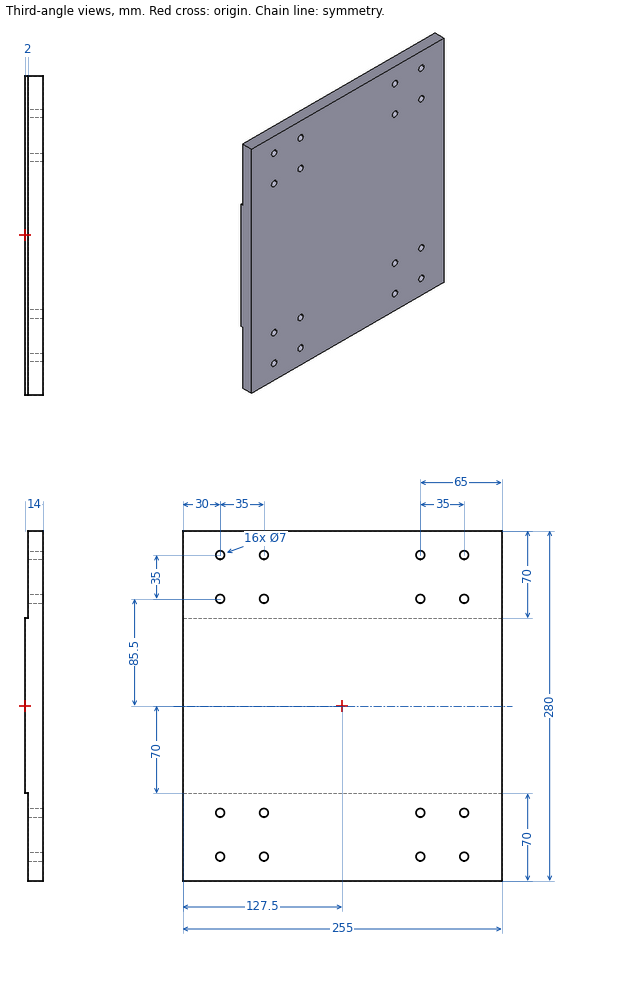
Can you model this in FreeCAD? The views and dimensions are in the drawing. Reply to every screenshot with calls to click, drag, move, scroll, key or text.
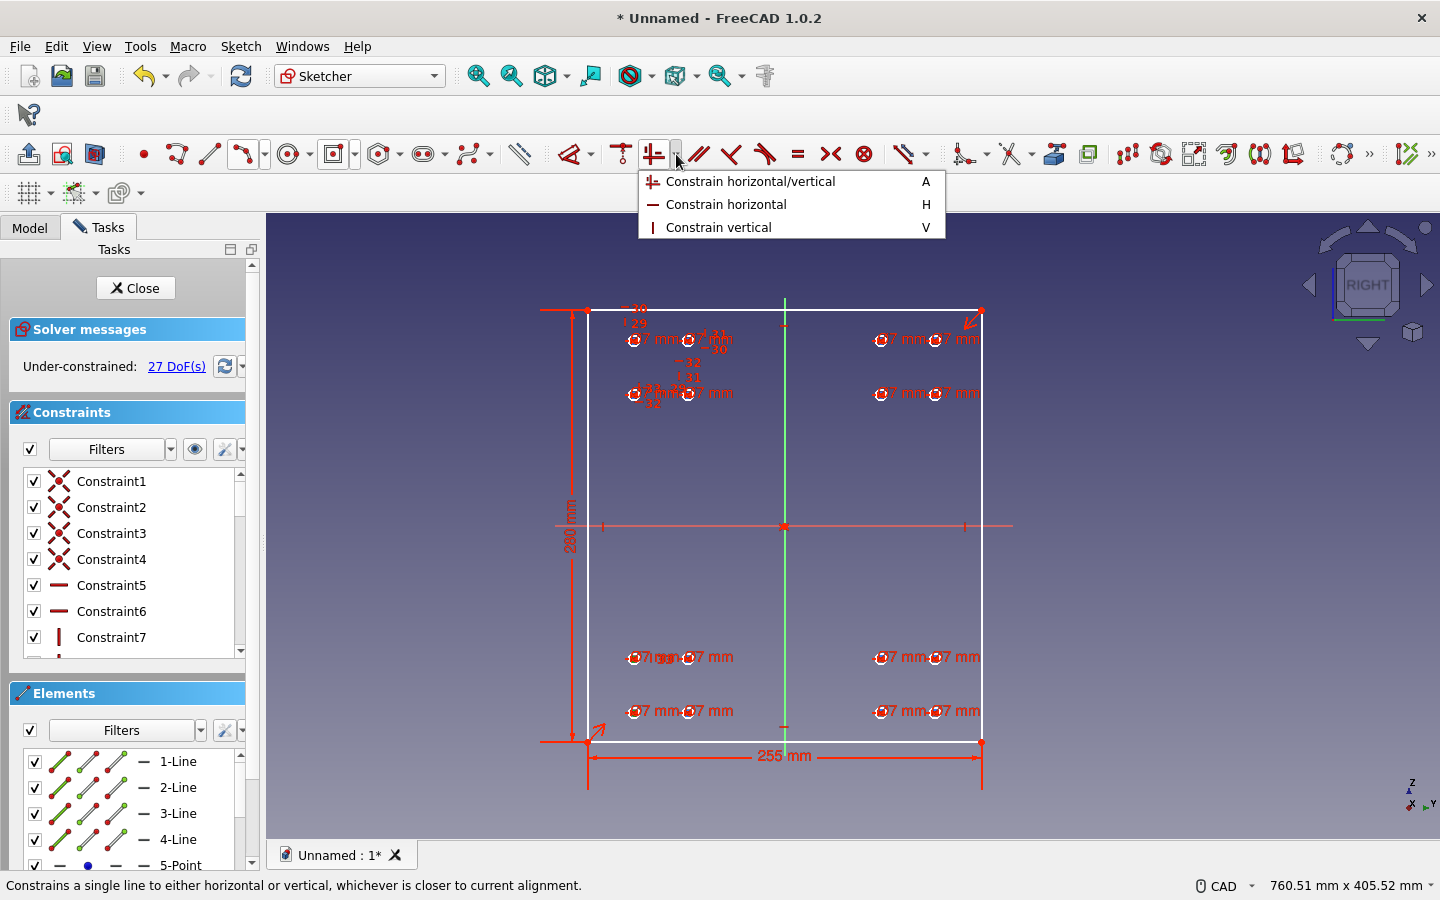
click(792, 228)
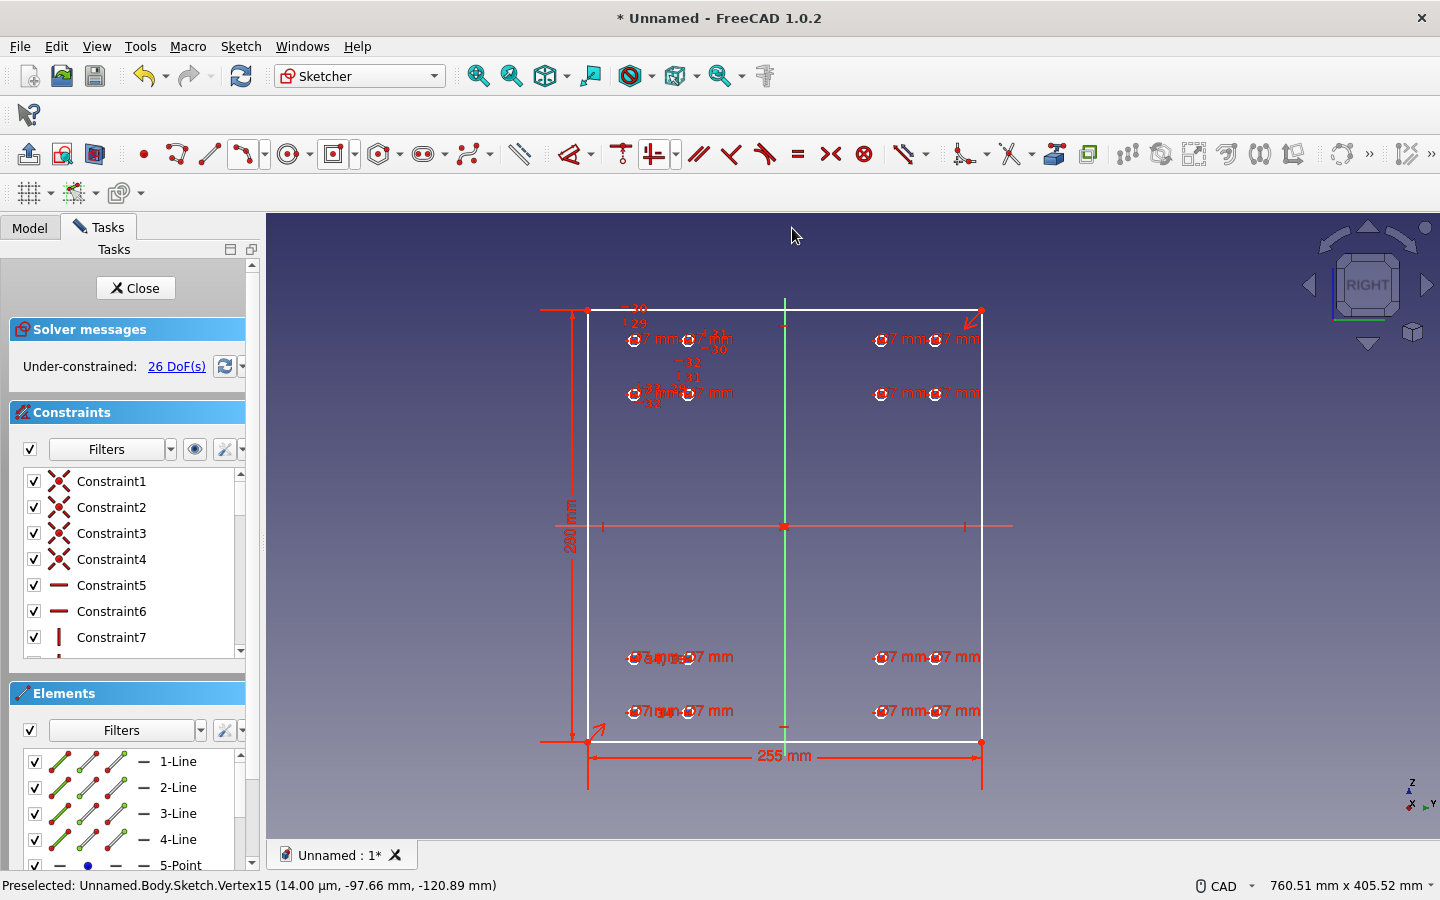
click(688, 395)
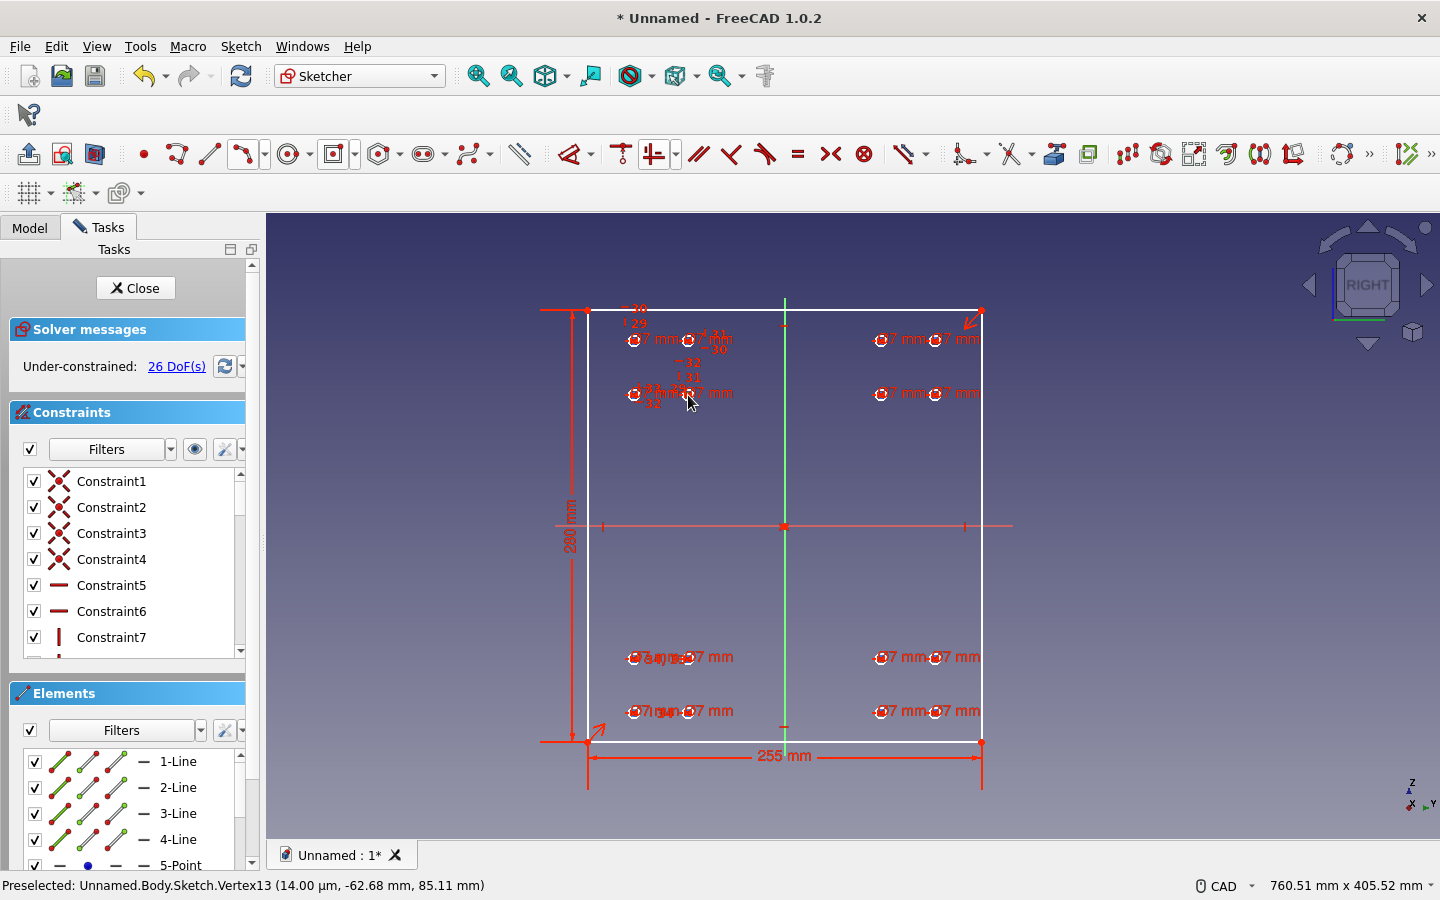
click(688, 659)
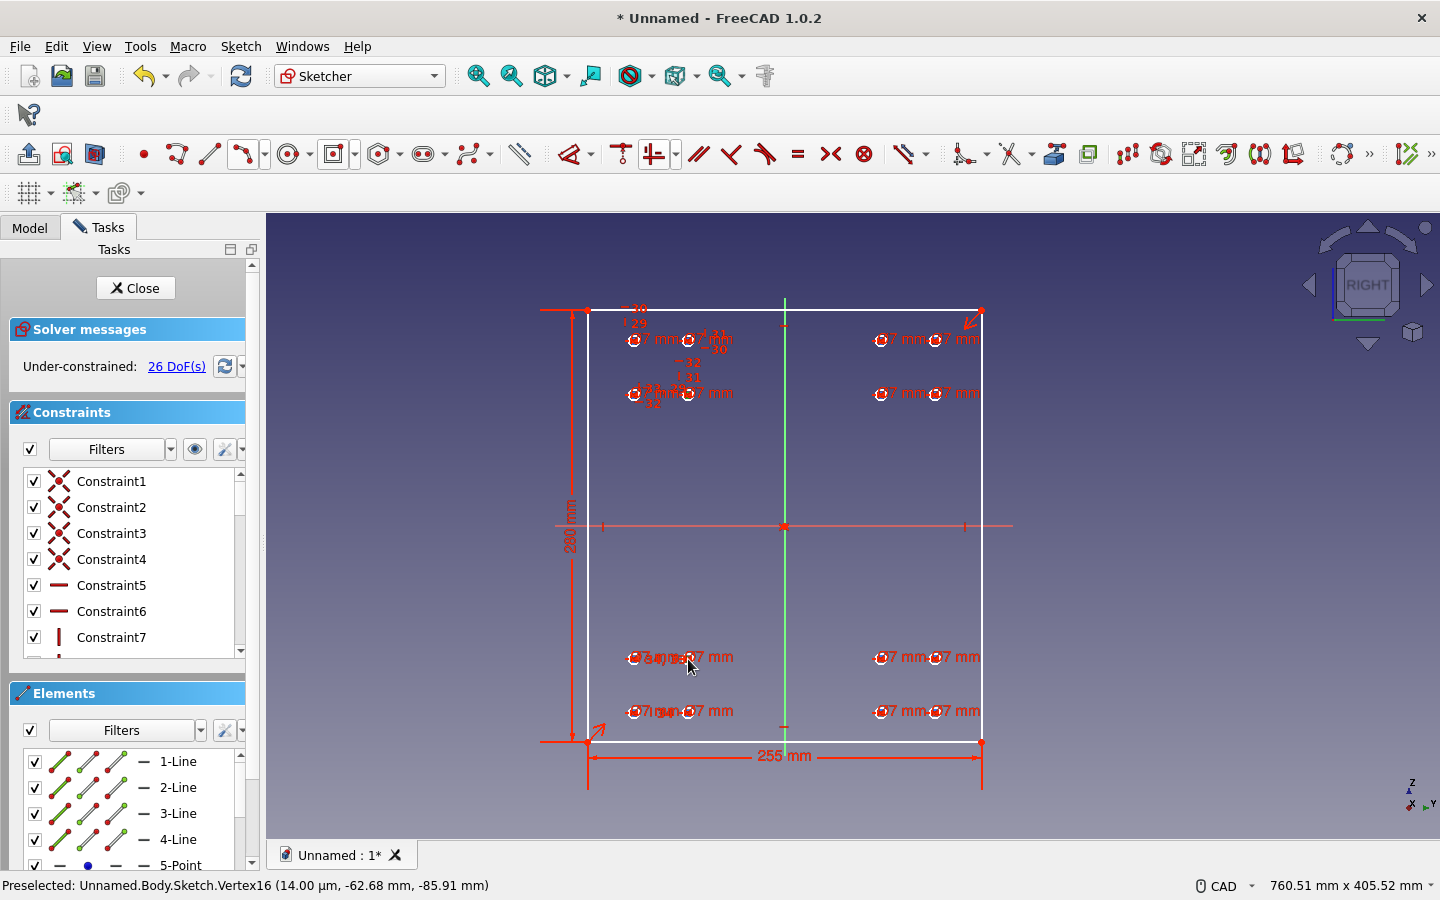
key(v)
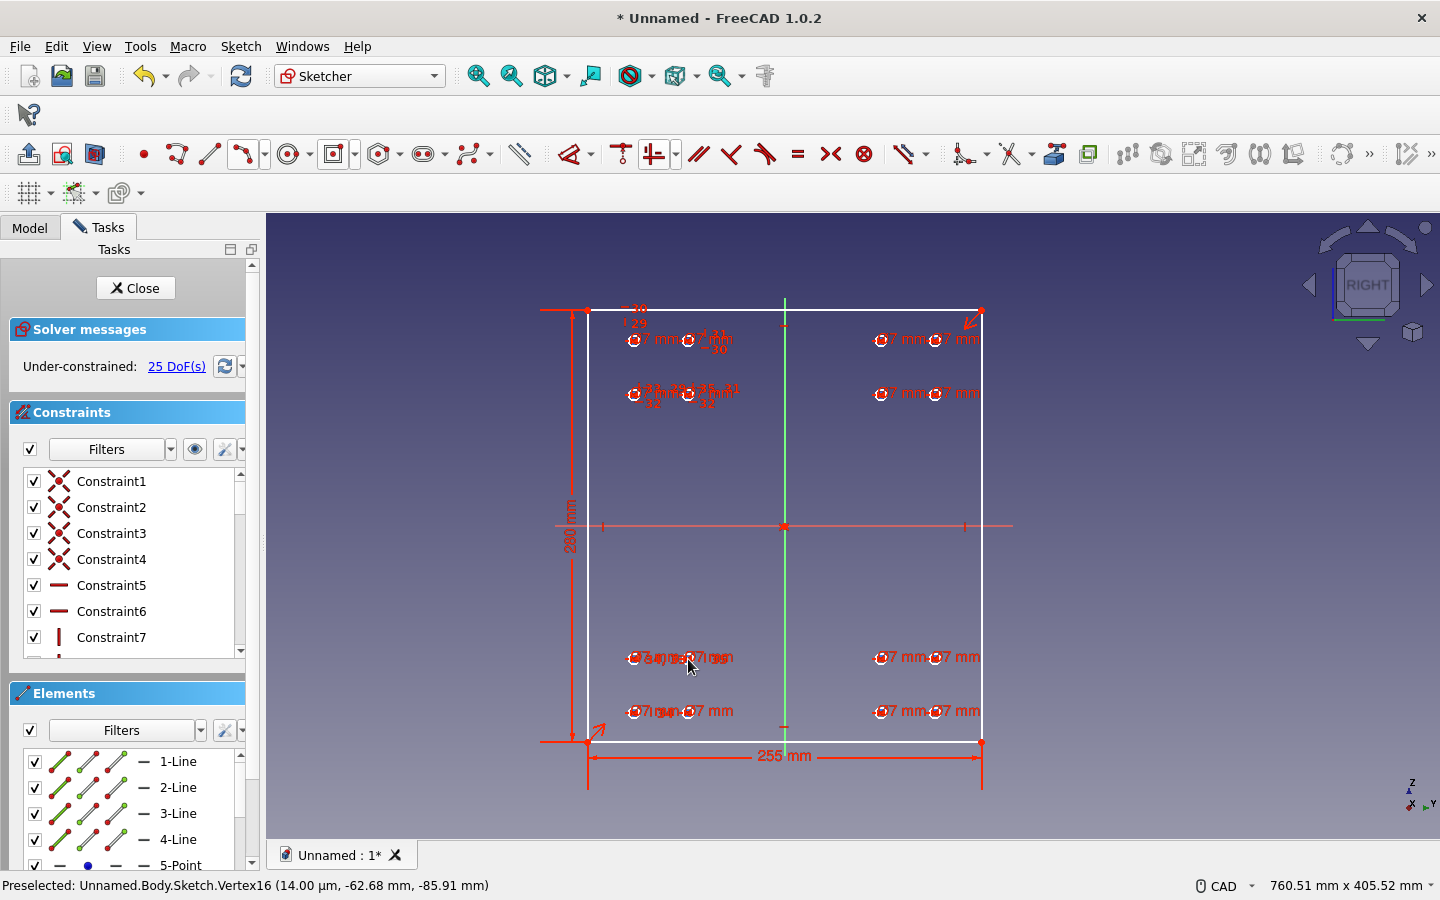
click(634, 659)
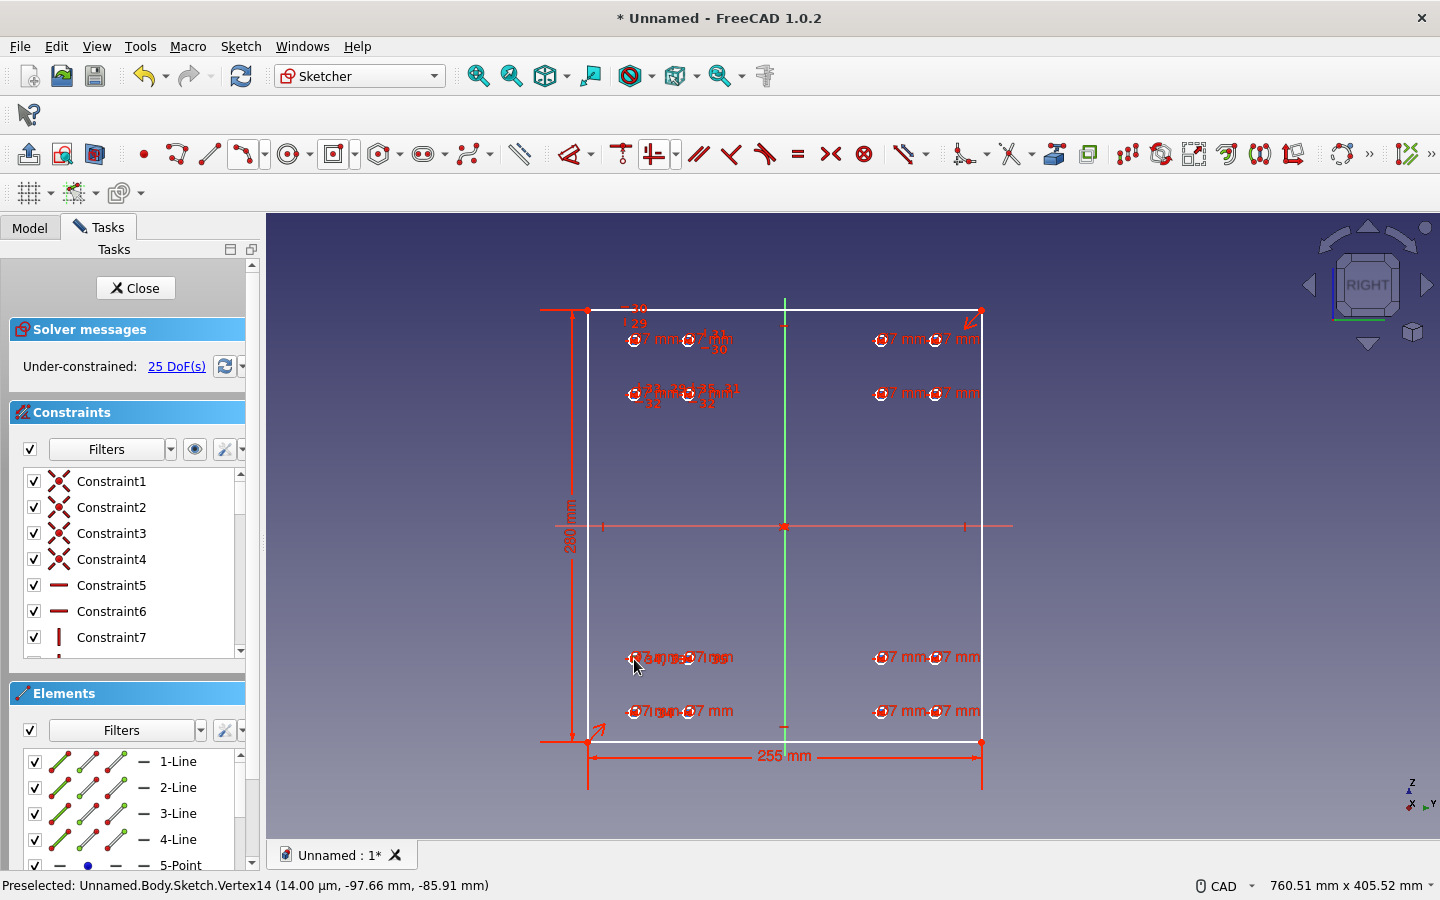
click(688, 659)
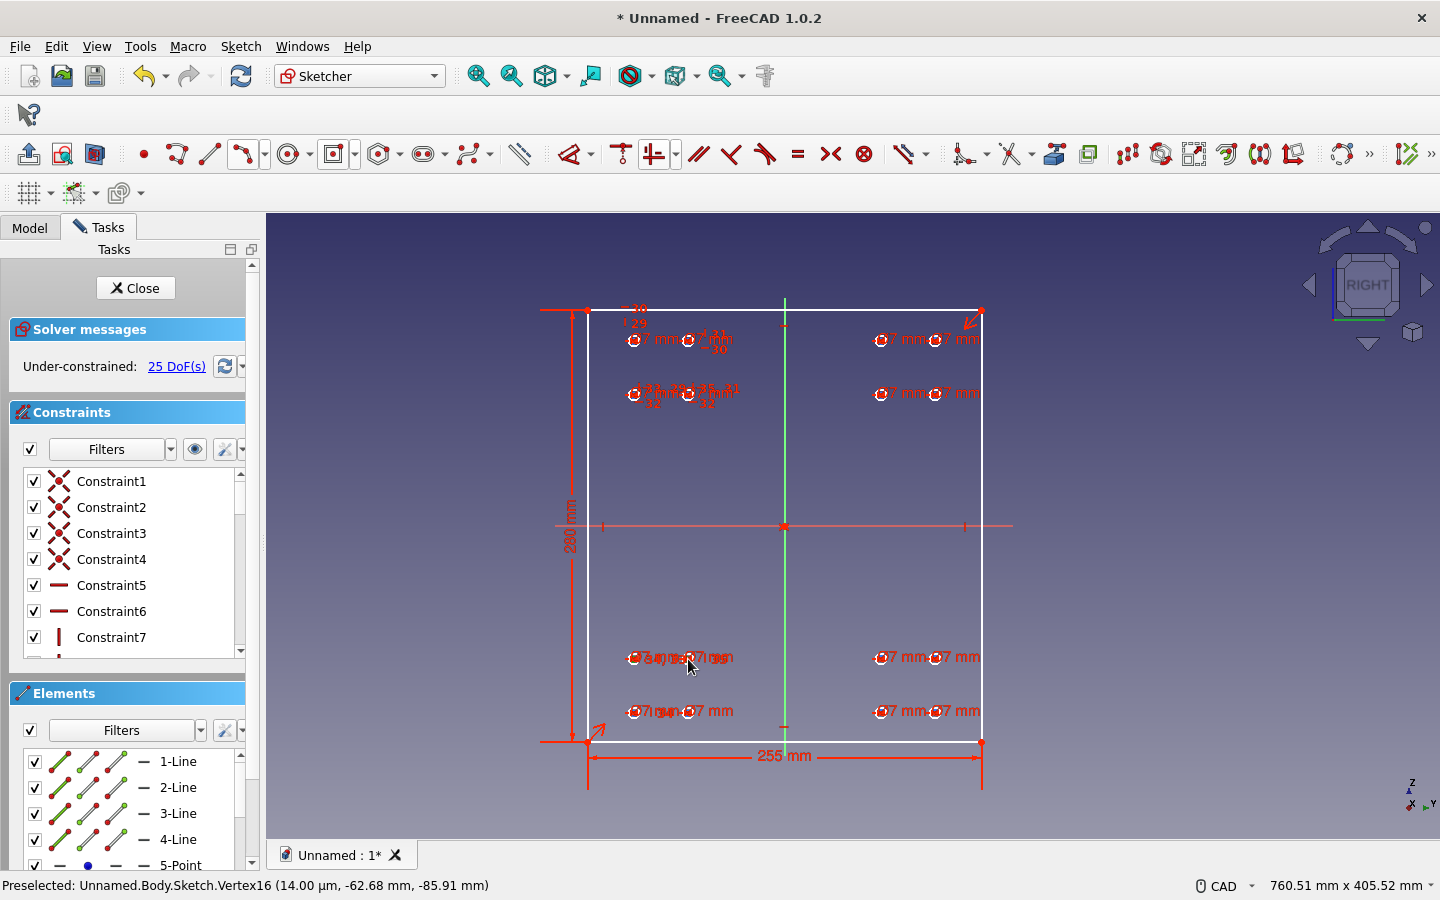
click(676, 154)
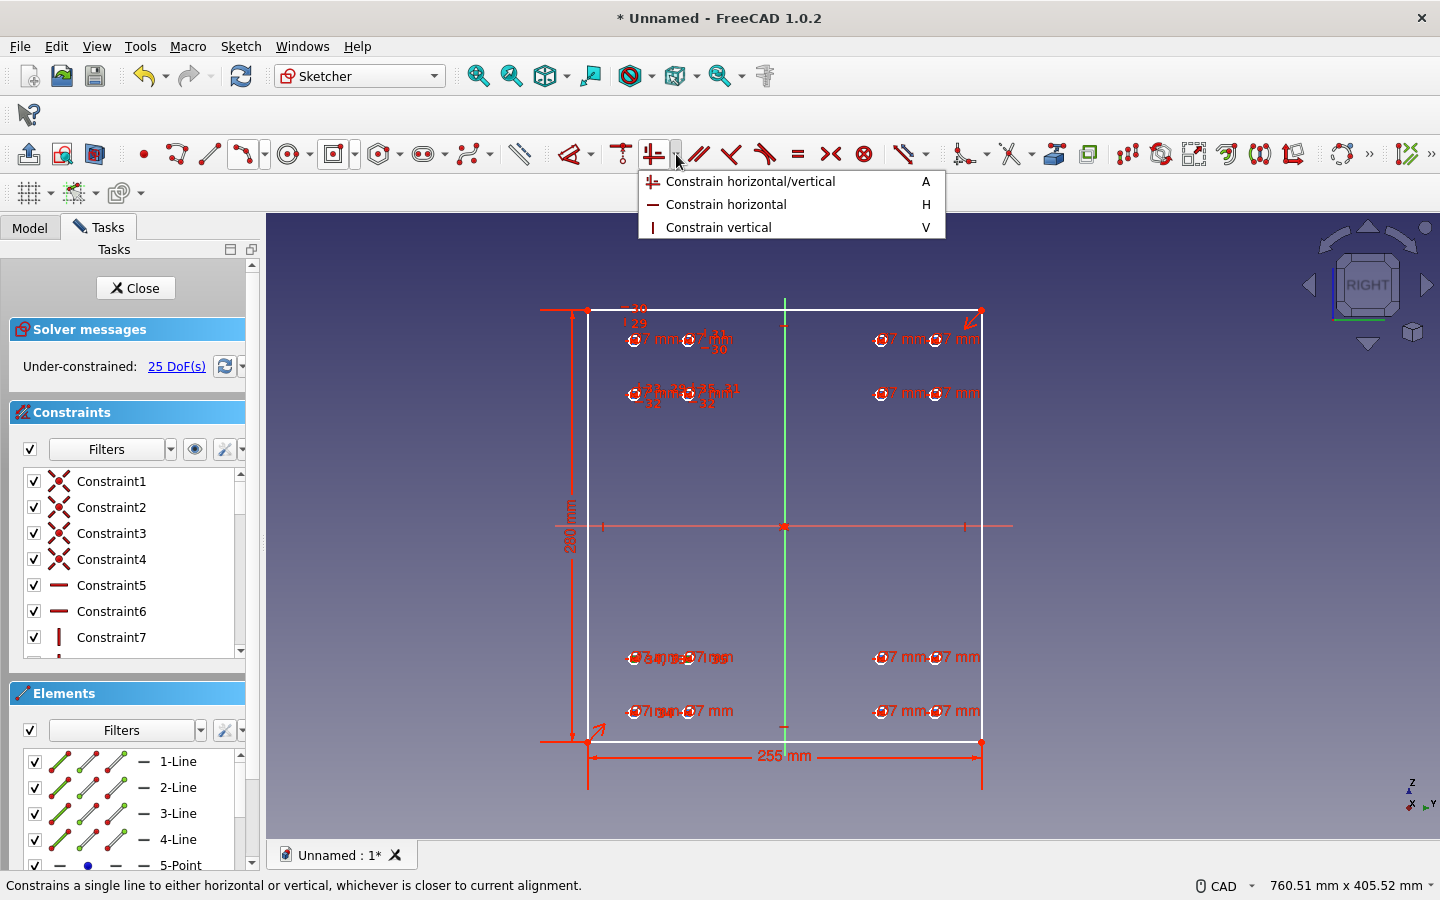
click(792, 204)